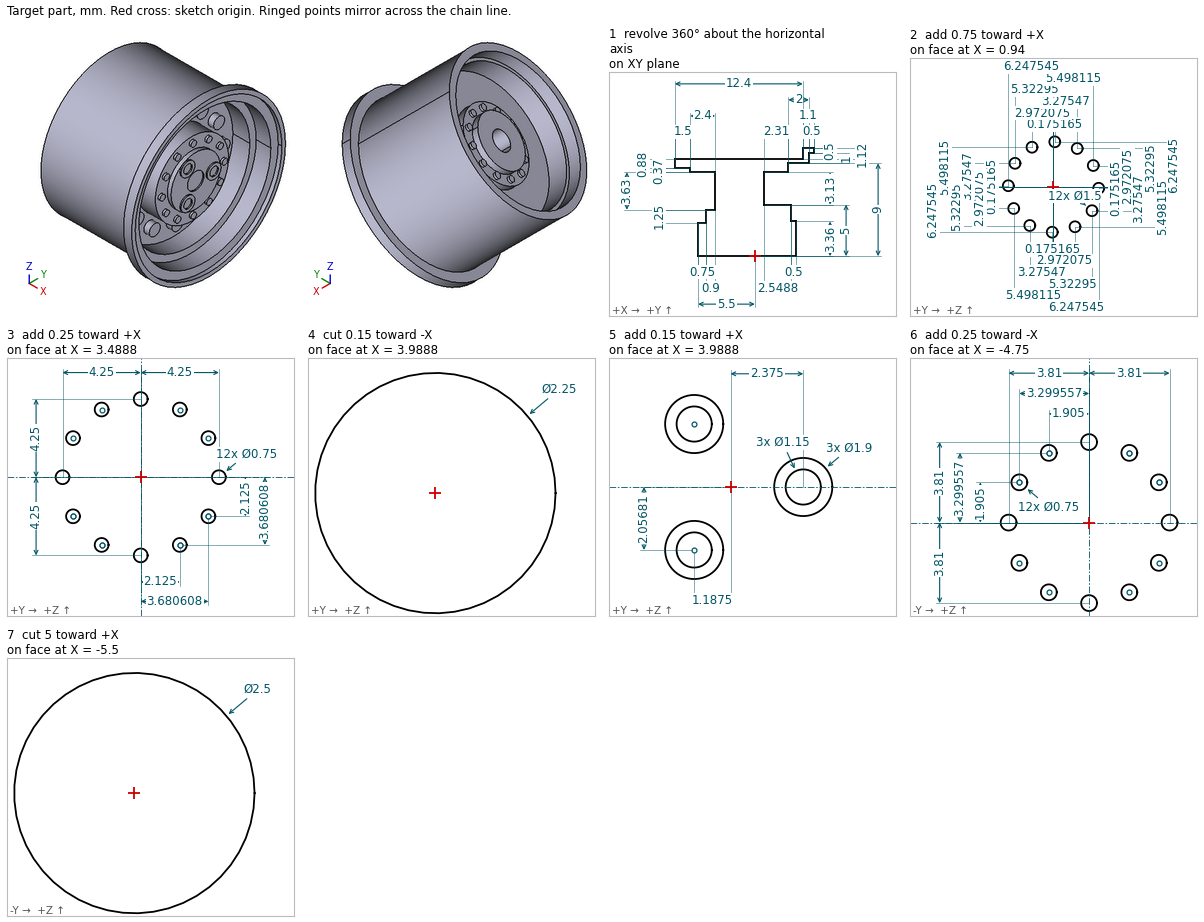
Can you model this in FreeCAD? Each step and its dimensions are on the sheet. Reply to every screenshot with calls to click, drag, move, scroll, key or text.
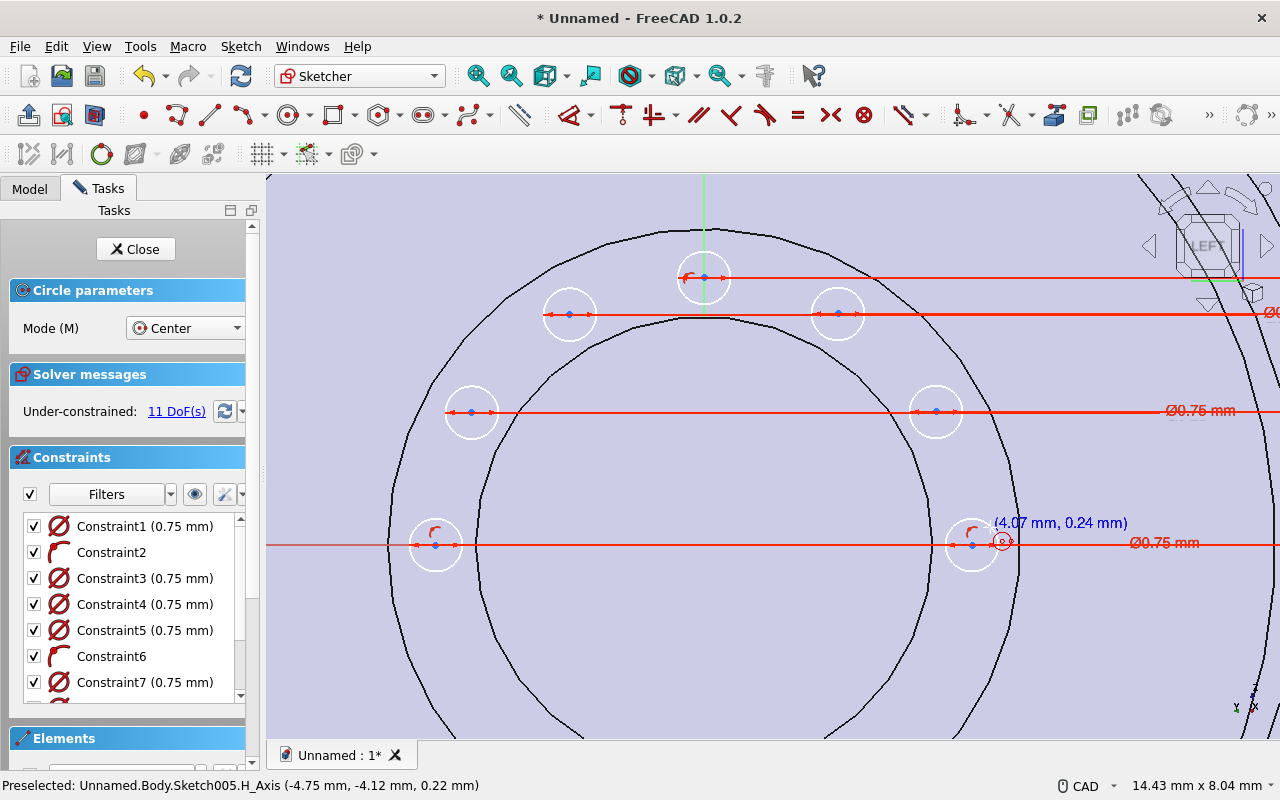
click(936, 679)
move(955, 660)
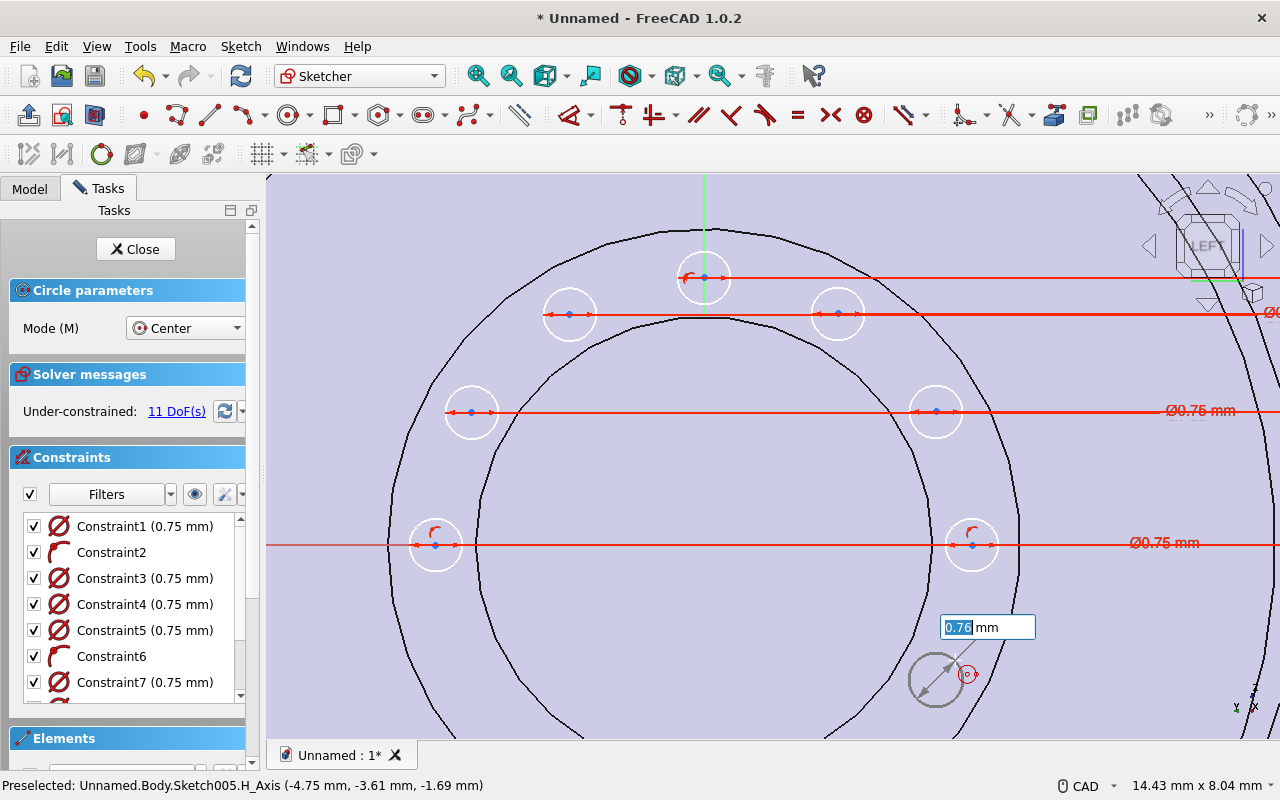
text(0.75)
key(Return)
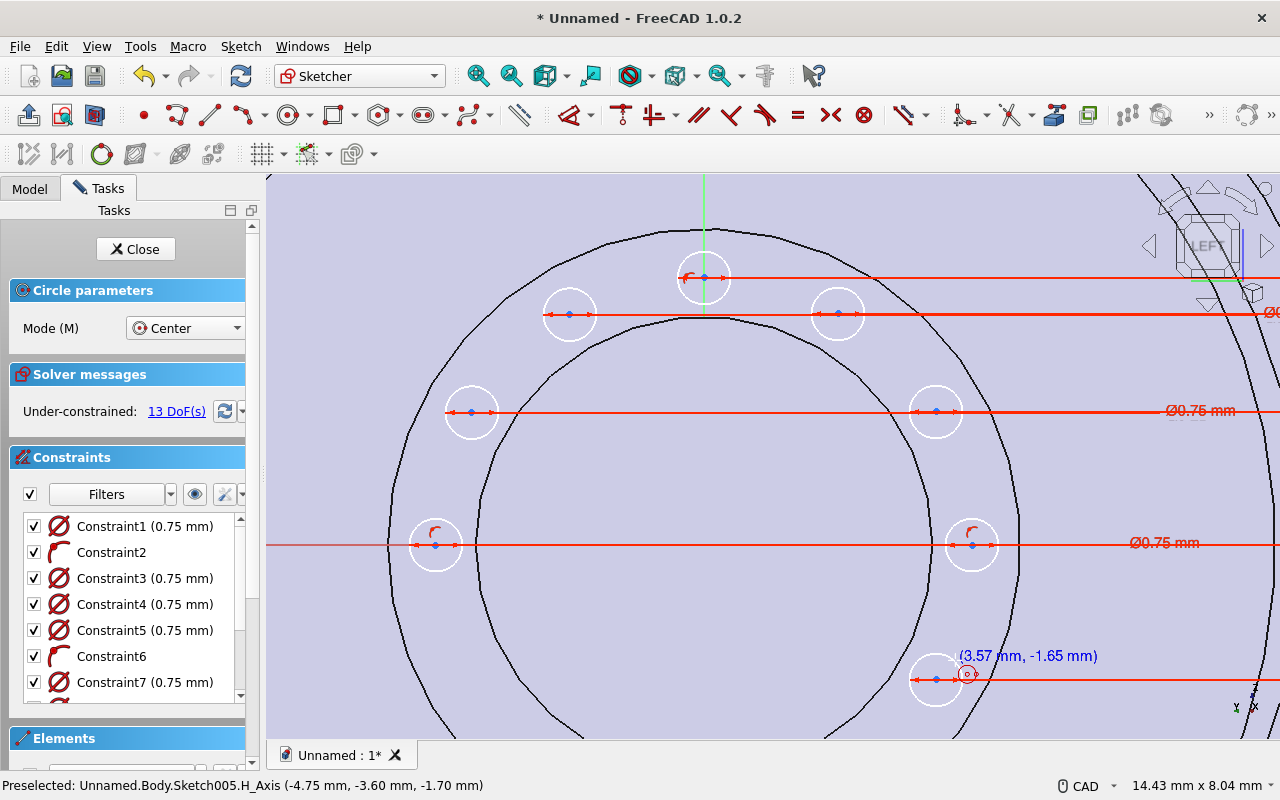
scroll(705, 276, down, 2)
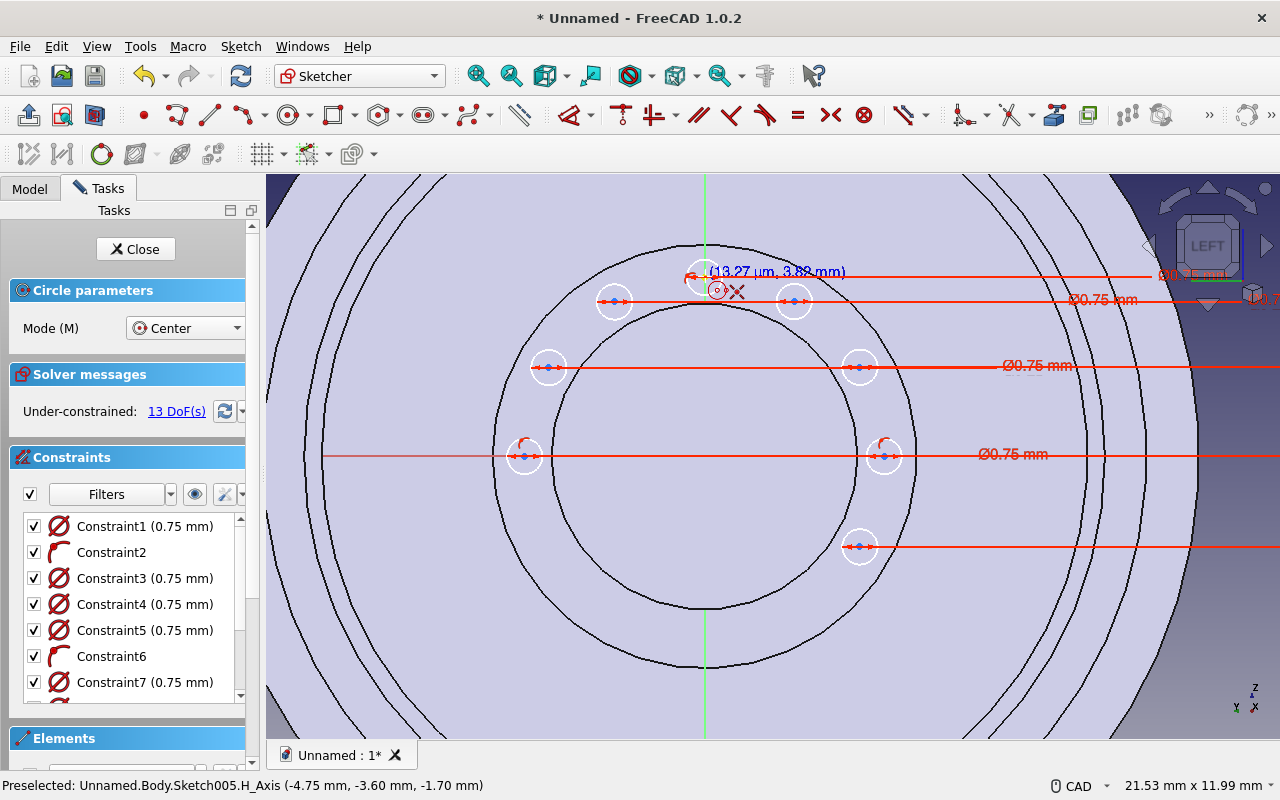
scroll(794, 612, up, 2)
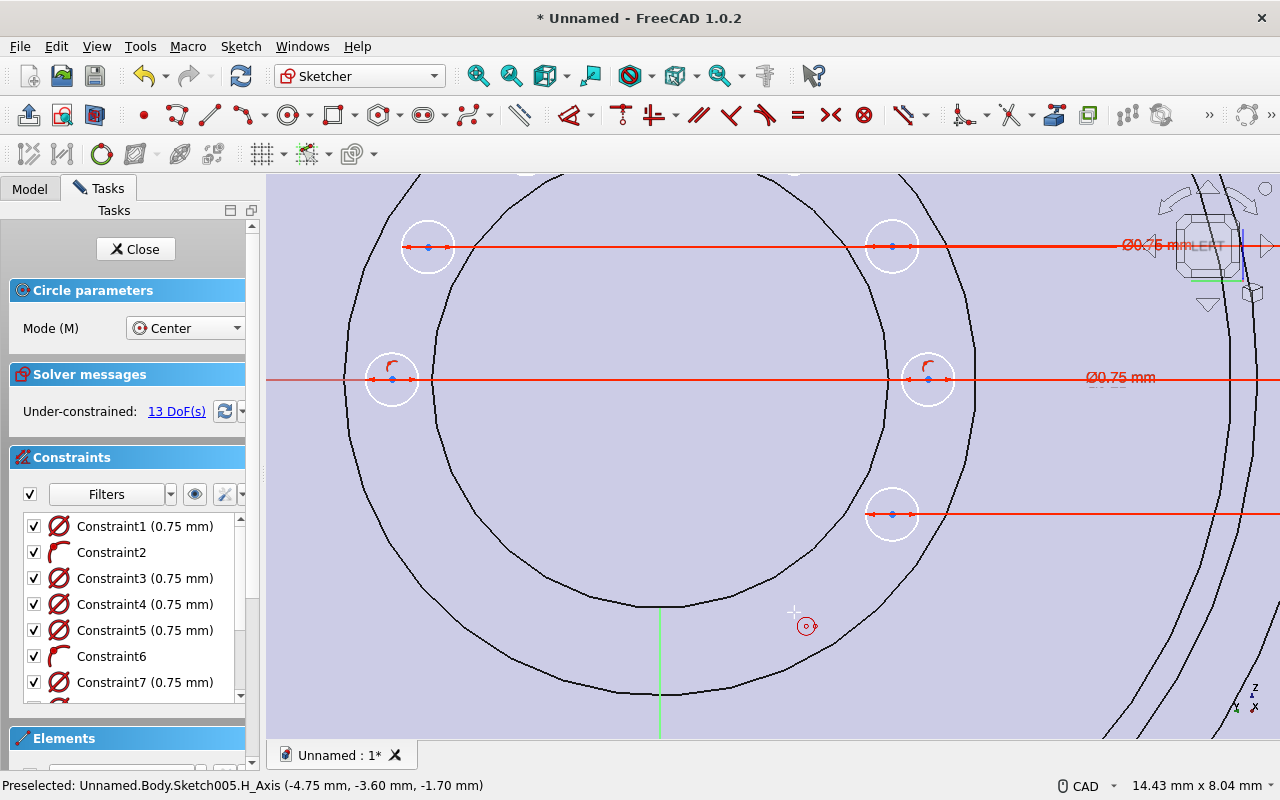
click(794, 611)
move(813, 593)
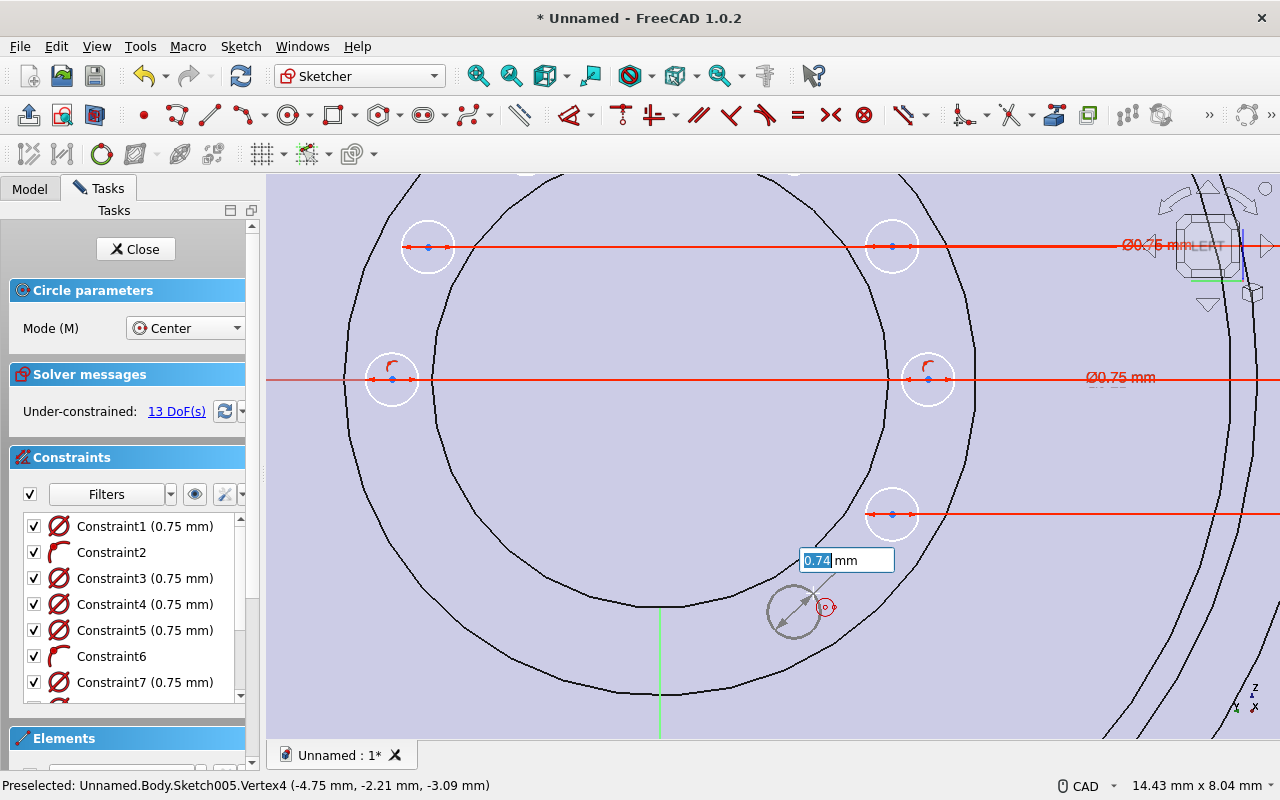
text(0.75)
key(Return)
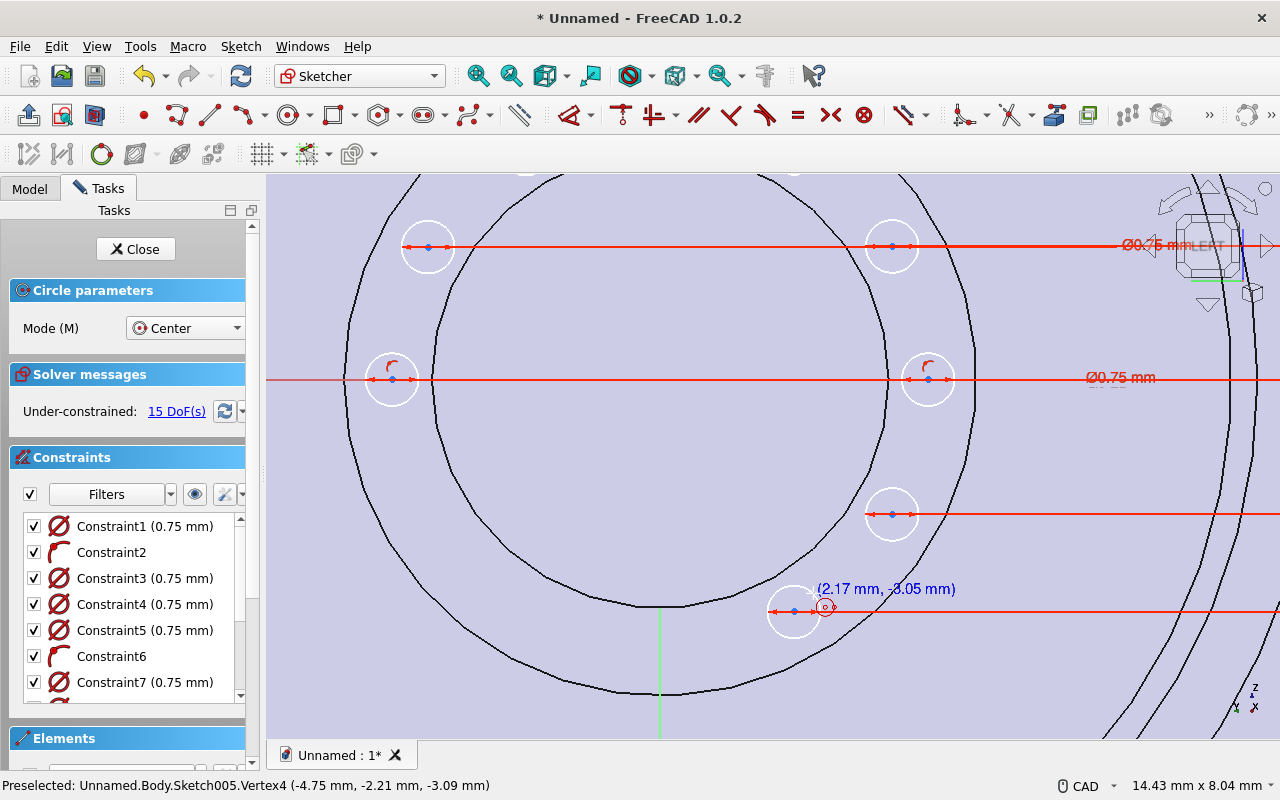
click(660, 647)
move(679, 629)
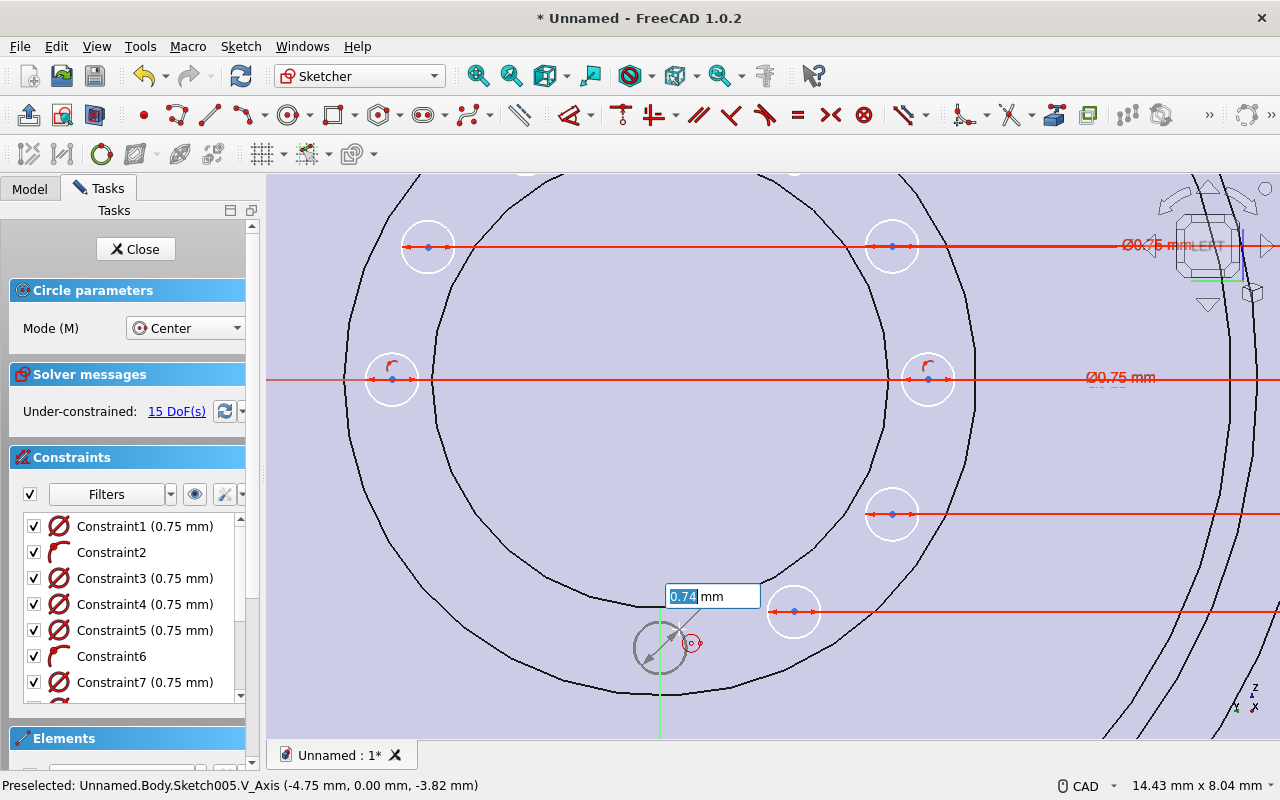
text(0.75)
key(Return)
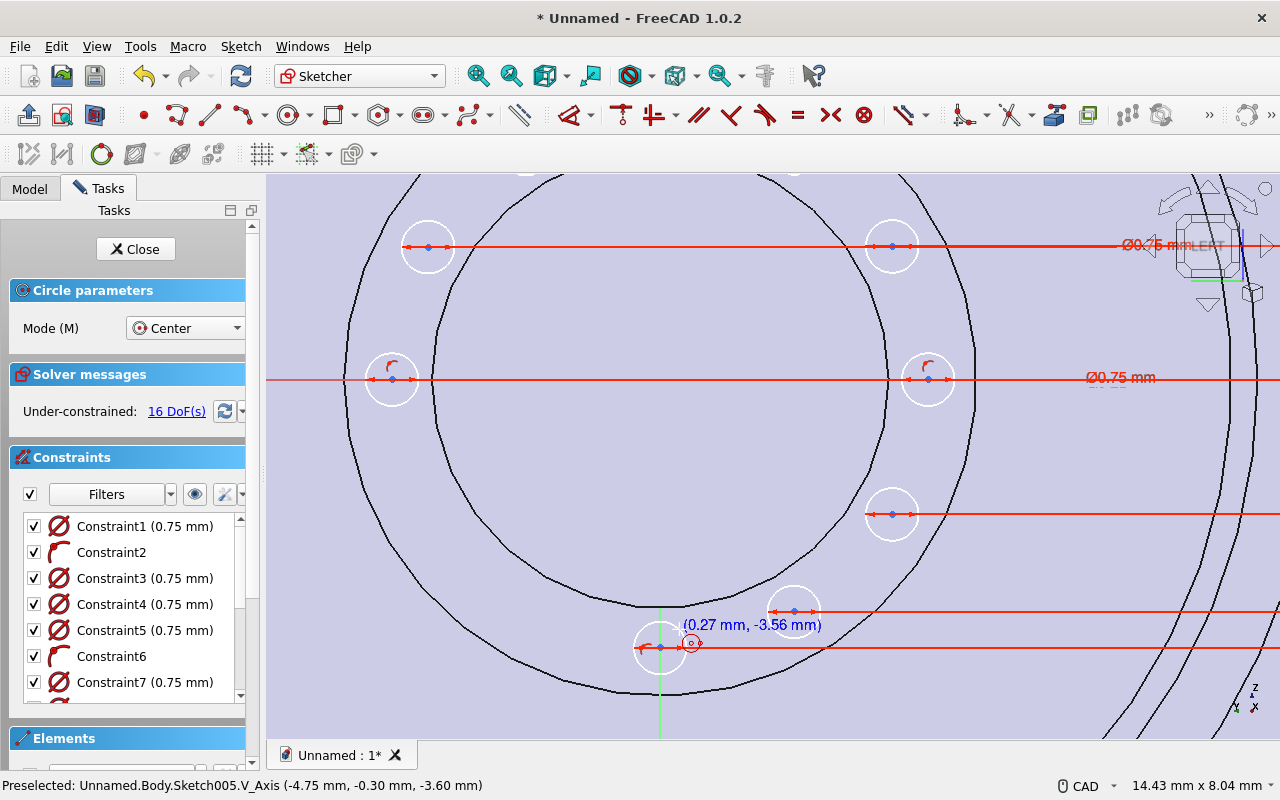
click(526, 611)
move(545, 593)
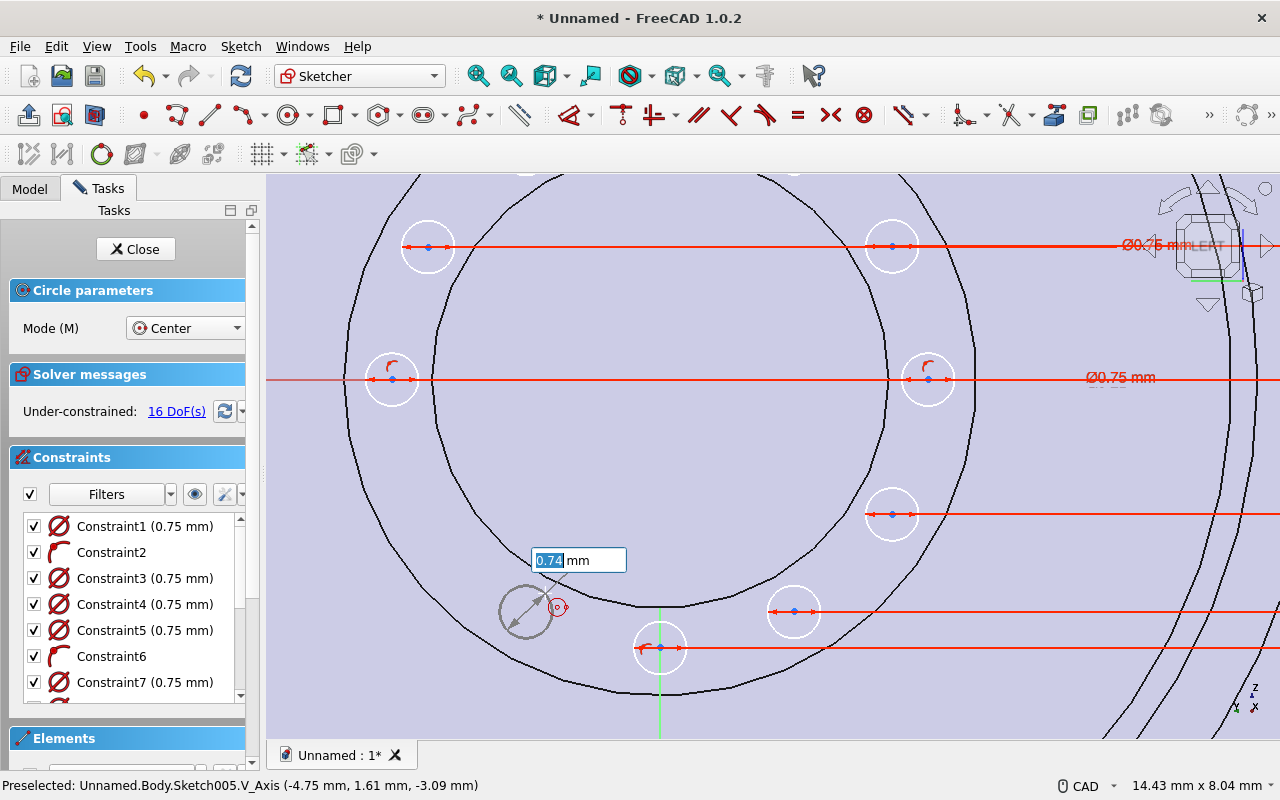
text(0.75)
key(Return)